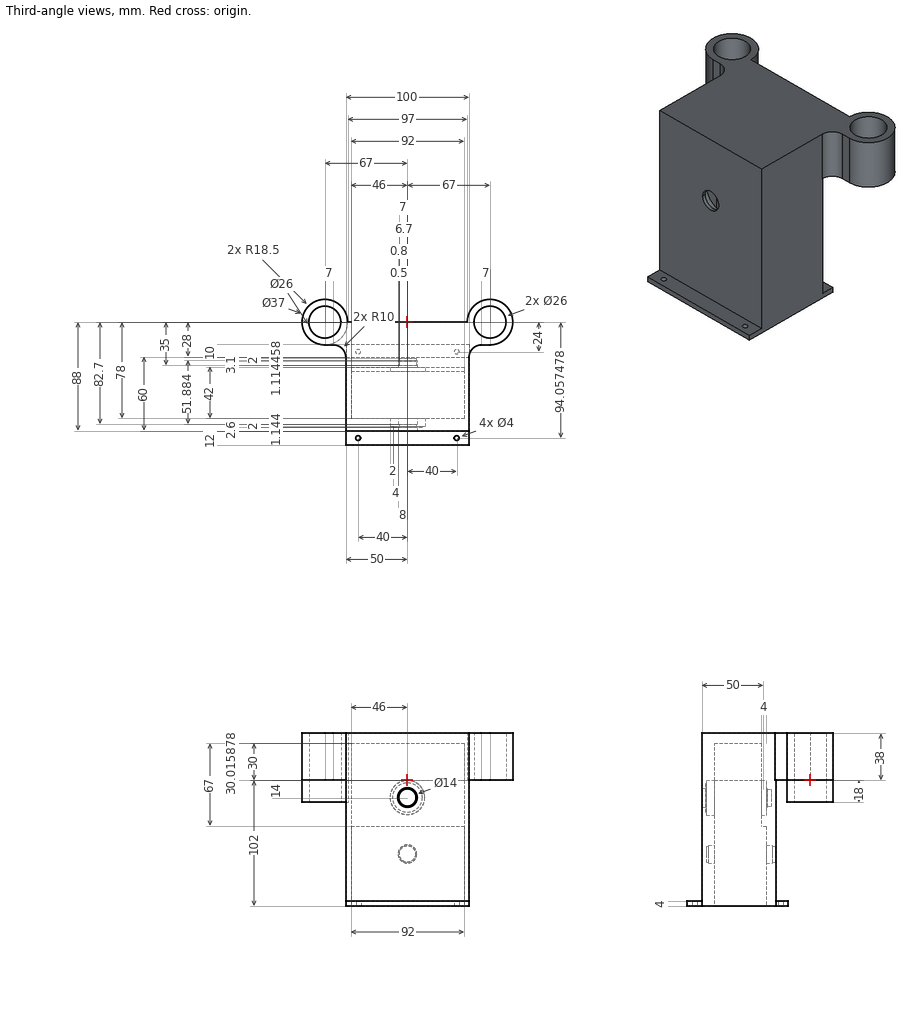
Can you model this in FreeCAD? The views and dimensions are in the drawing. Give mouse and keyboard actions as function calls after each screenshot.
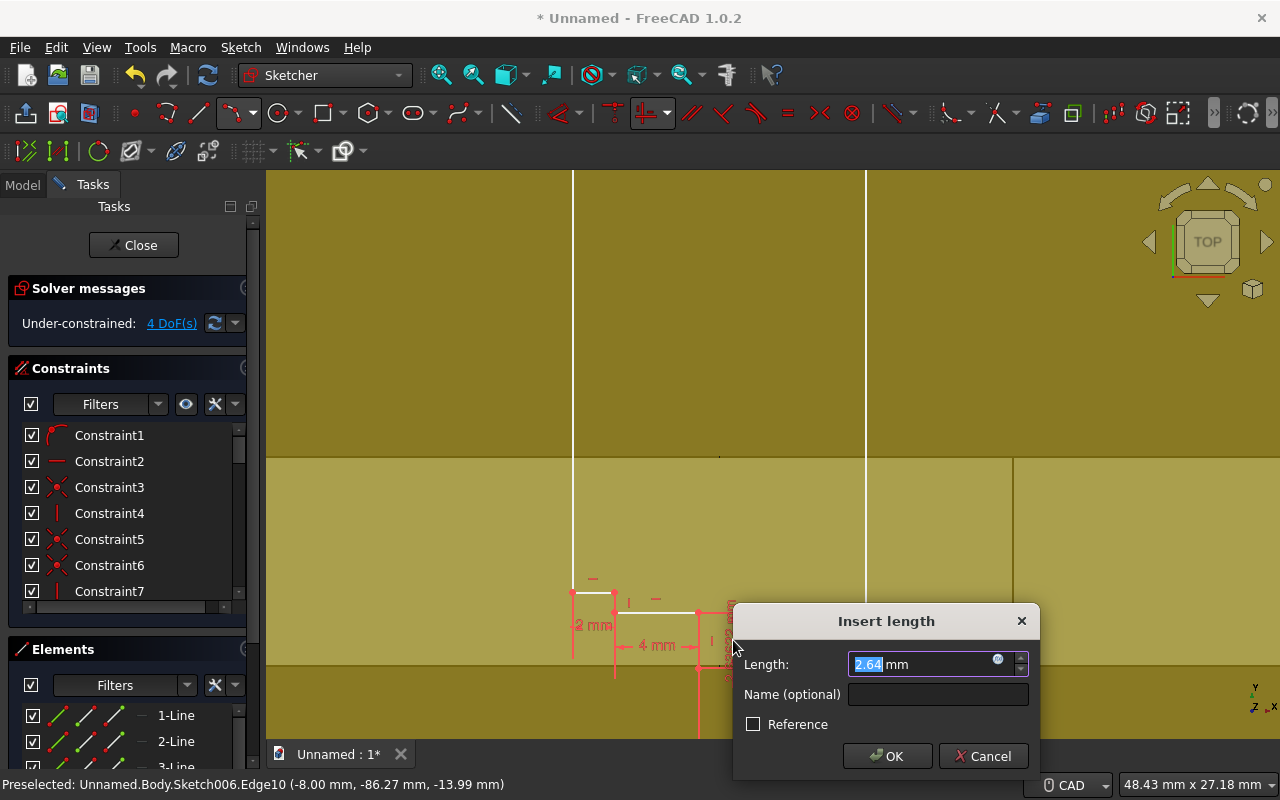
text(2.6)
key(Return)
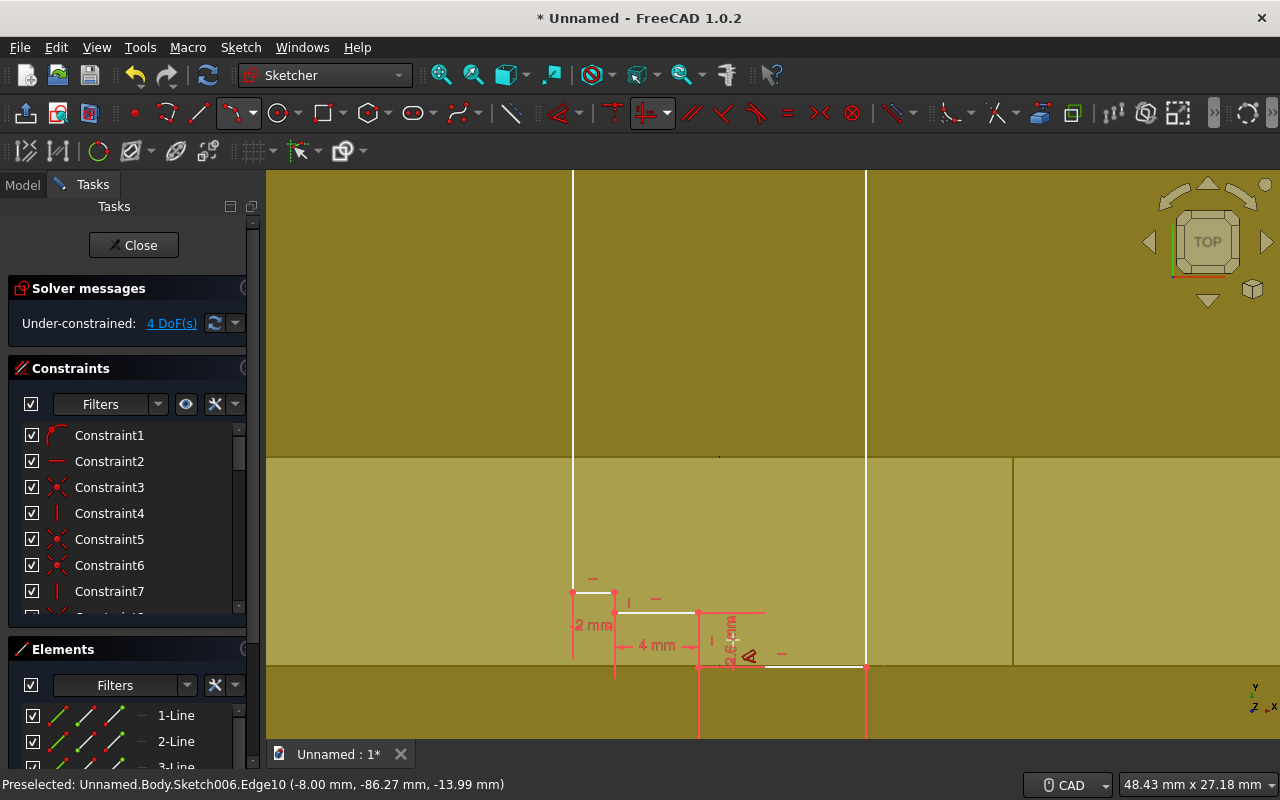
scroll(701, 634, down, 8)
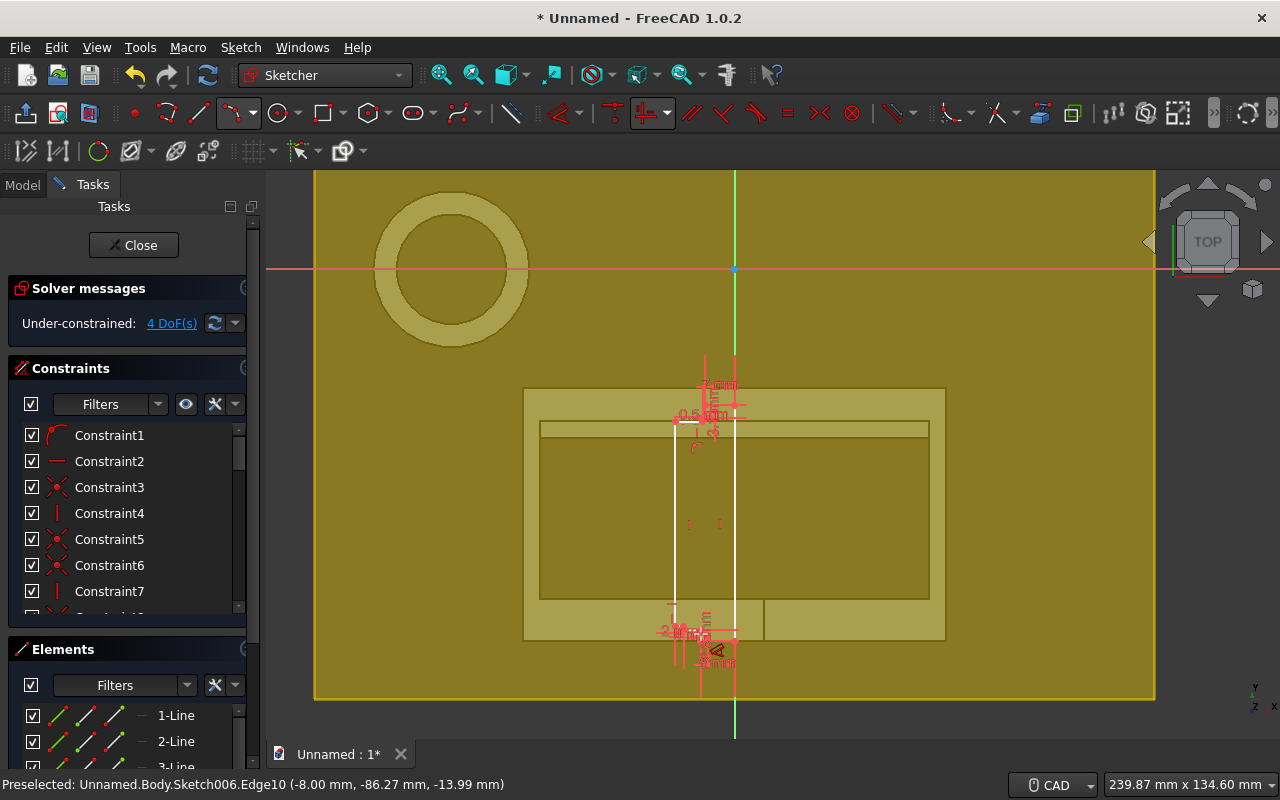
scroll(705, 418, up, 9)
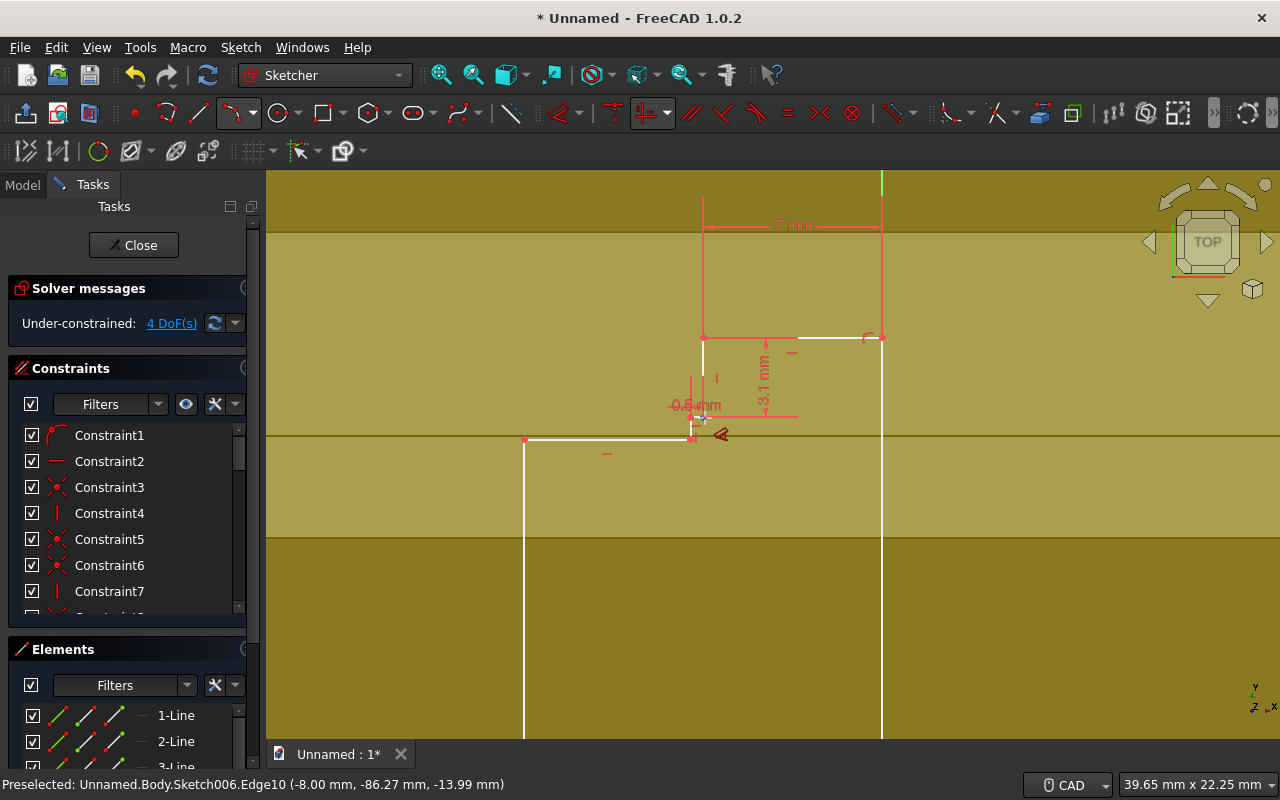
click(703, 417)
click(916, 308)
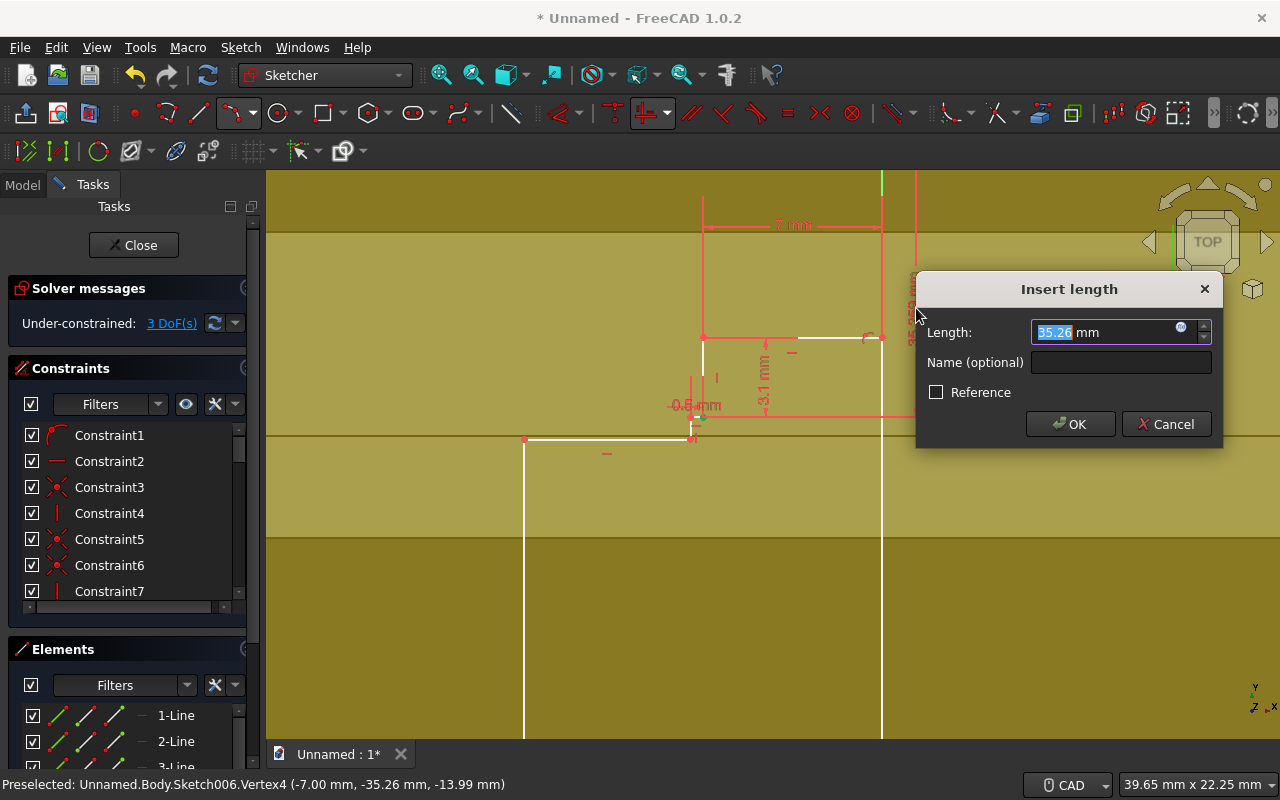
text(35)
key(Return)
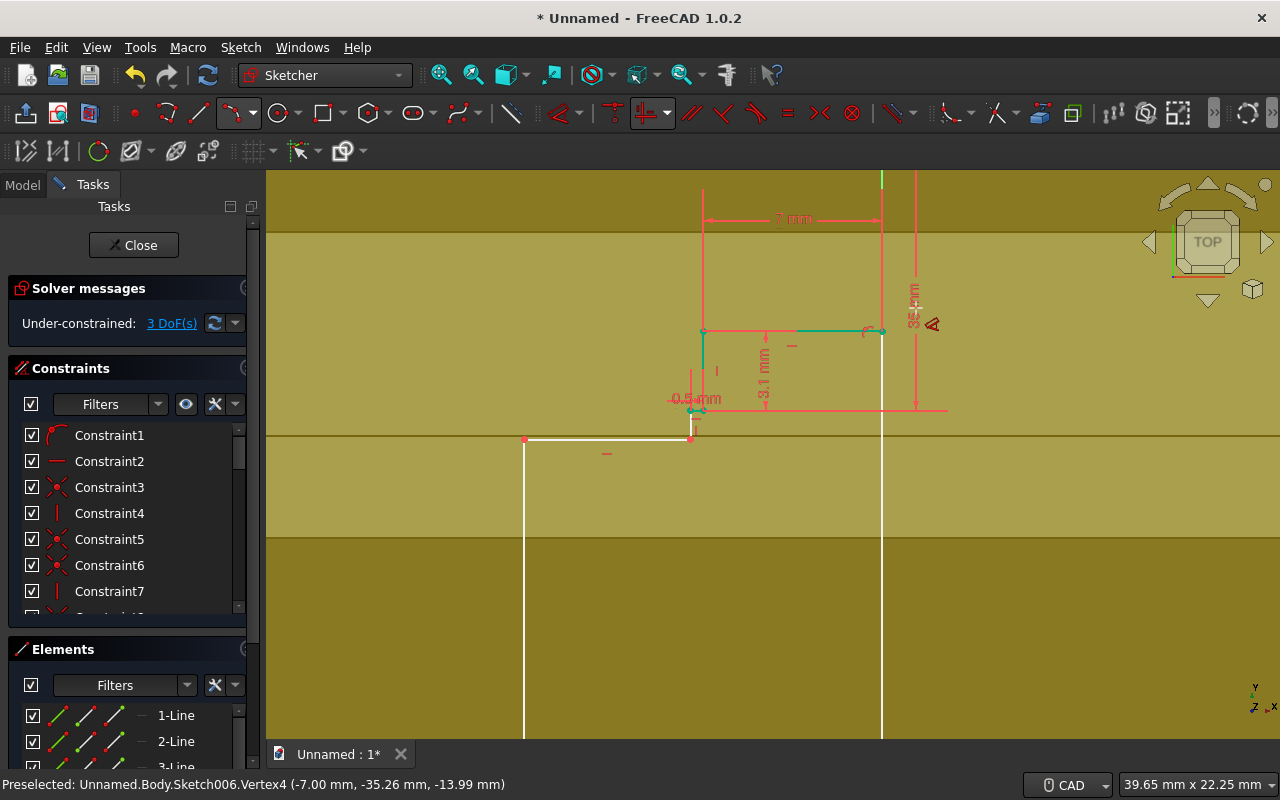
scroll(705, 418, down, 9)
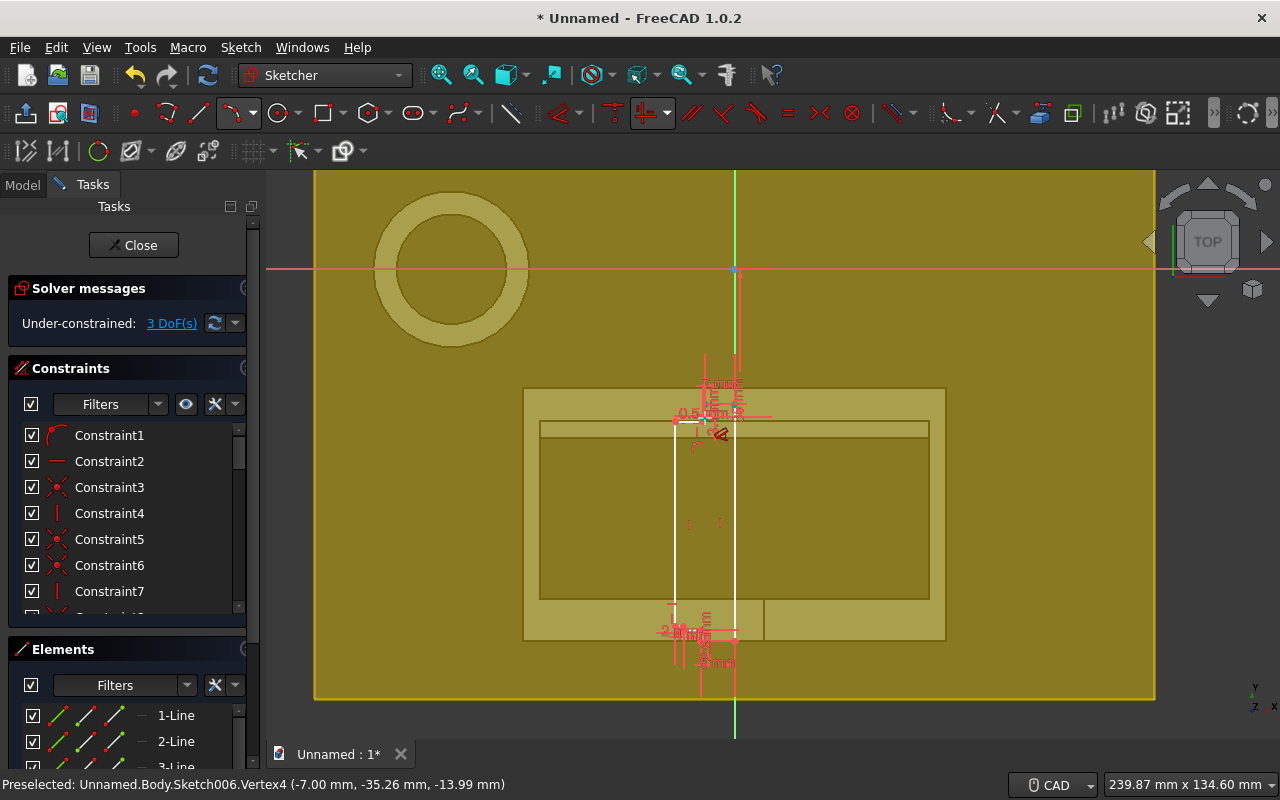
click(701, 641)
click(769, 455)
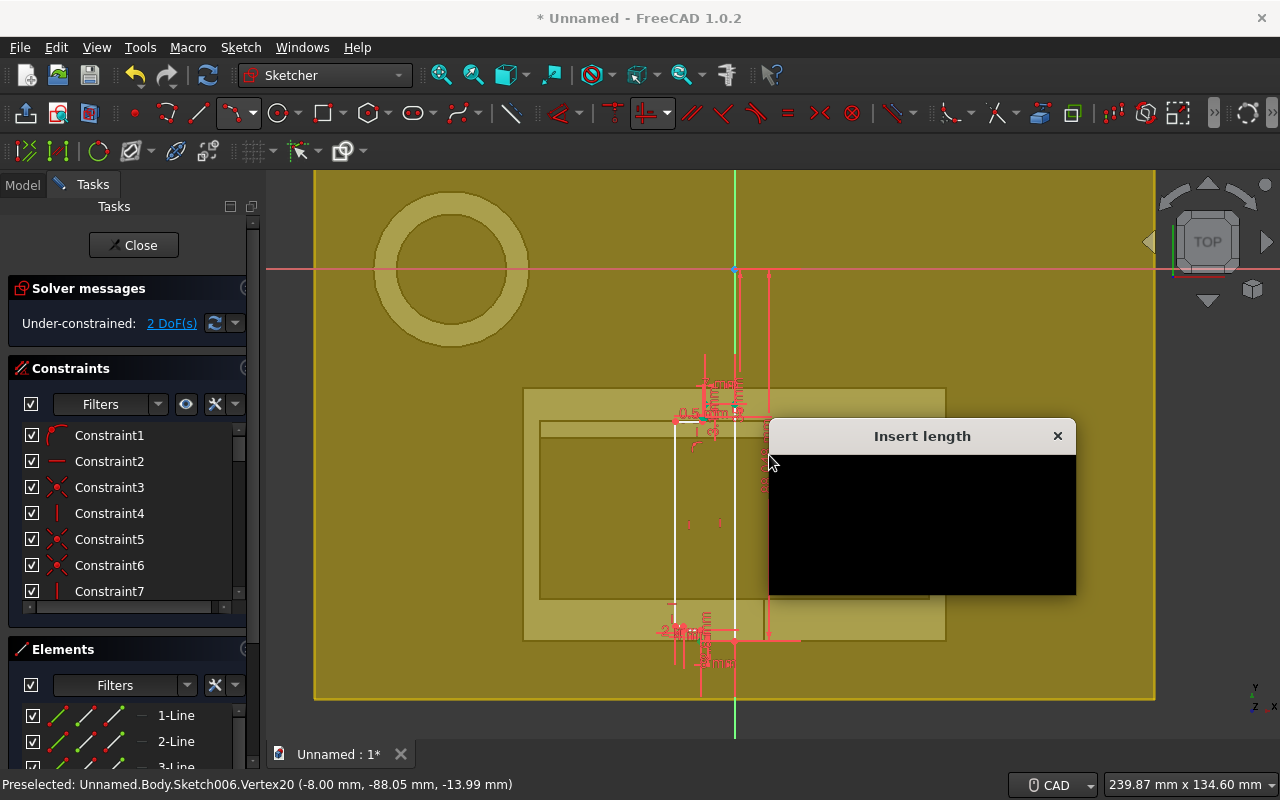
text(88)
key(Return)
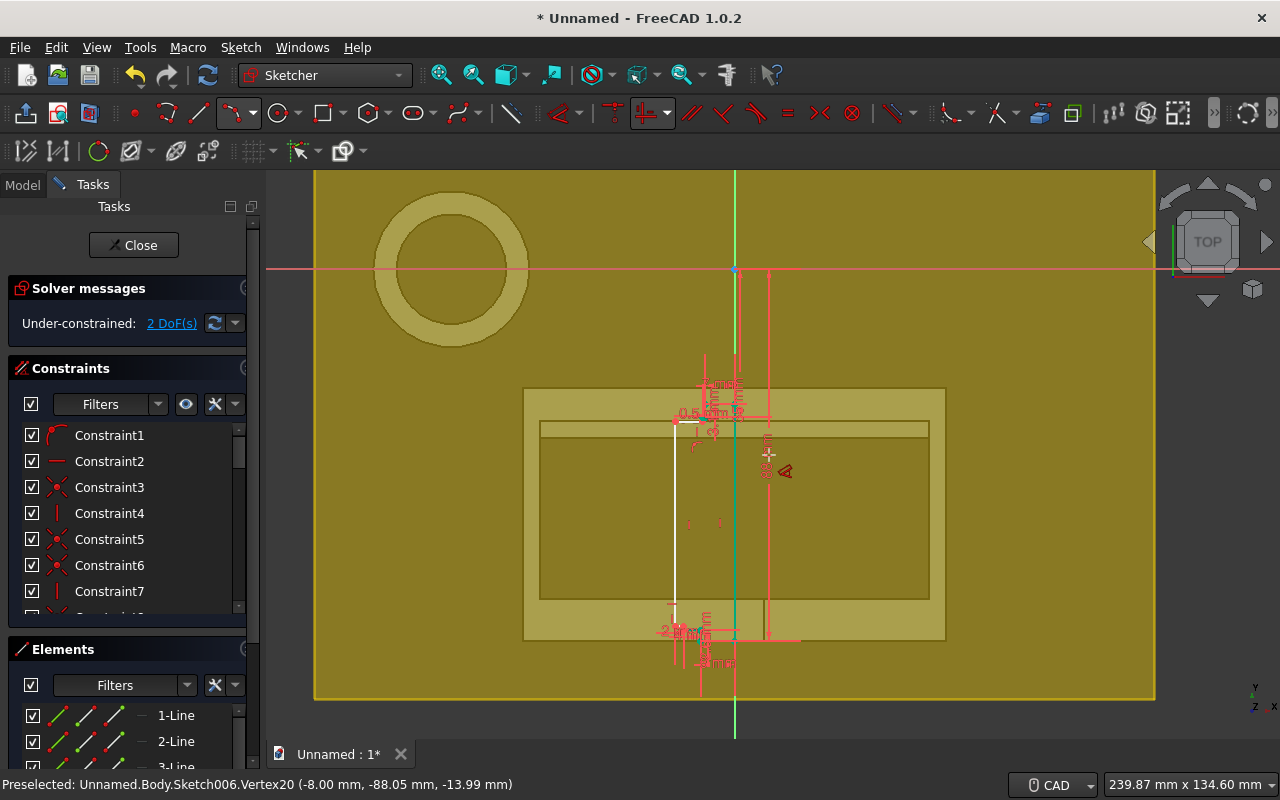
scroll(684, 628, up, 11)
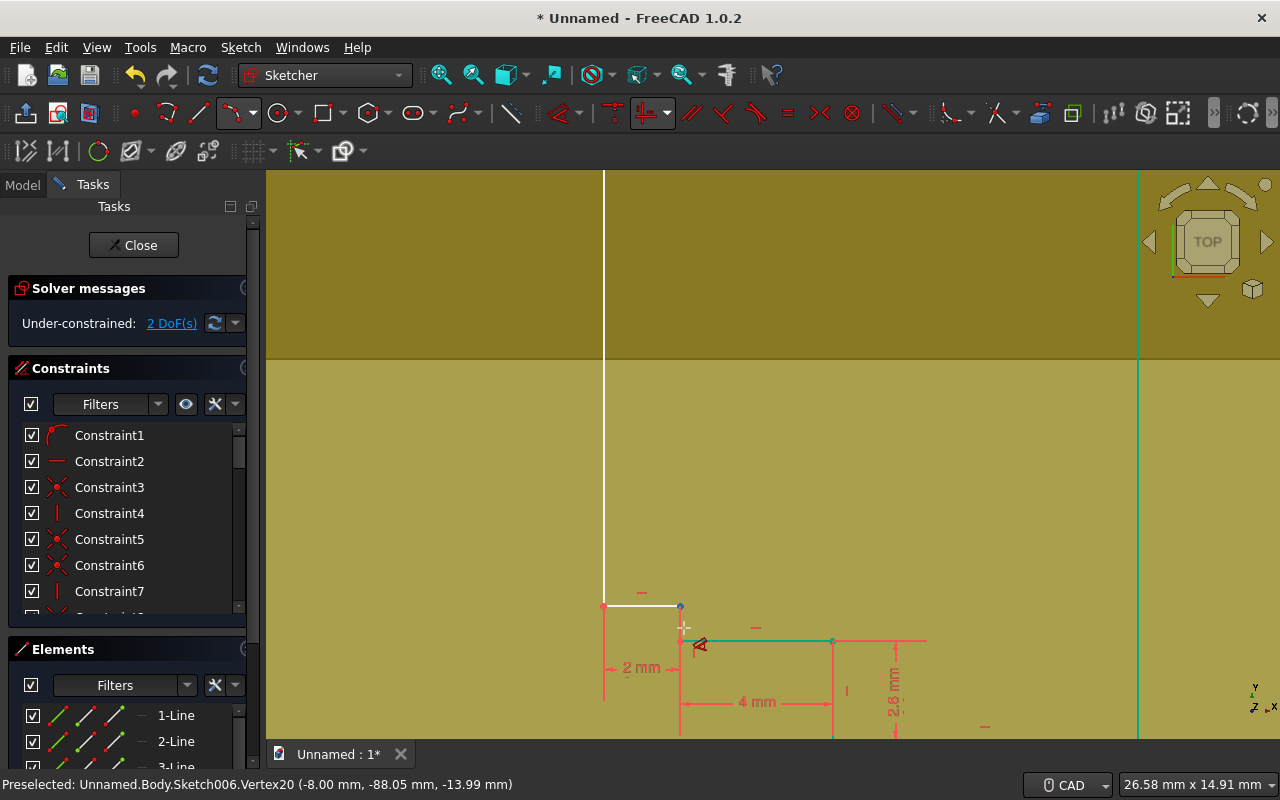
click(680, 624)
click(646, 624)